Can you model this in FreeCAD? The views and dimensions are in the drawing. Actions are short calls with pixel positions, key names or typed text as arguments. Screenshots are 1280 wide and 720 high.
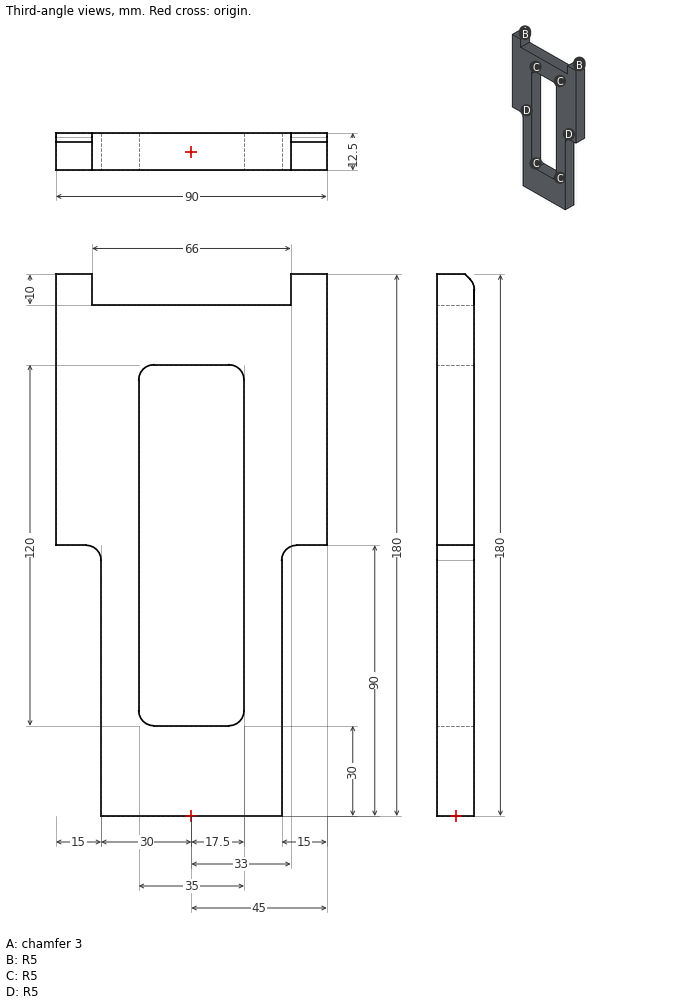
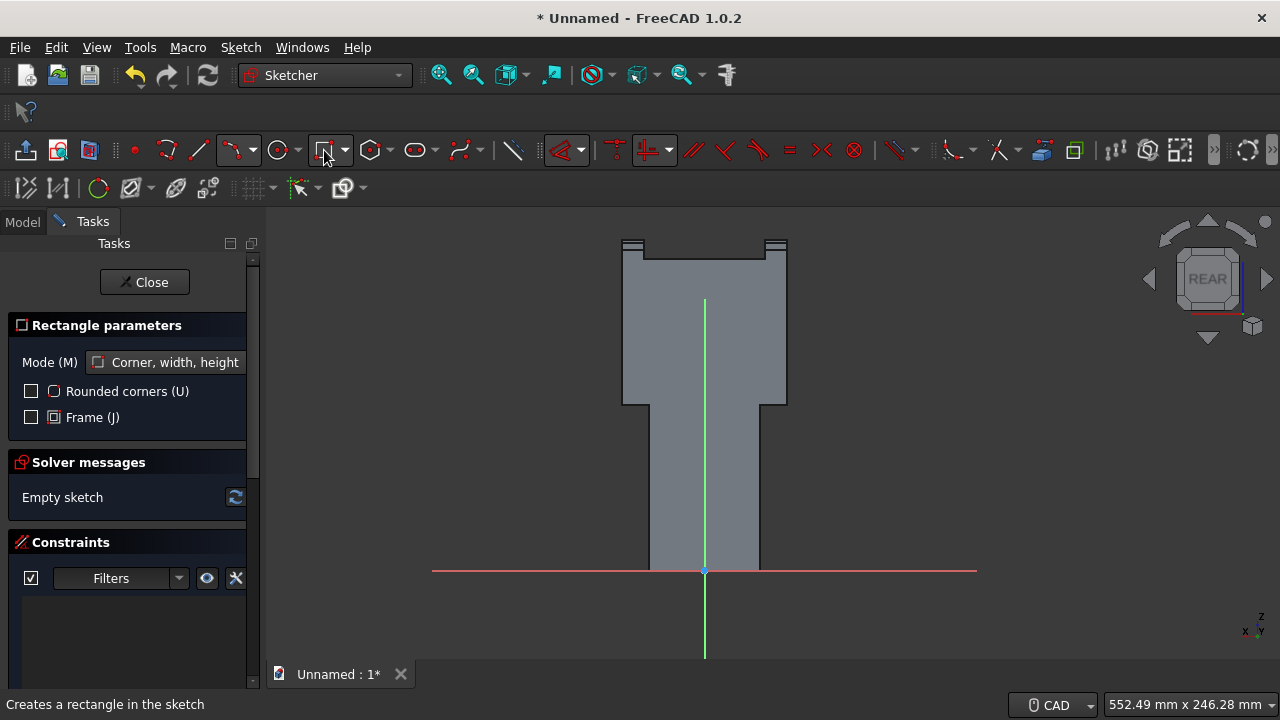
click(672, 295)
move(737, 516)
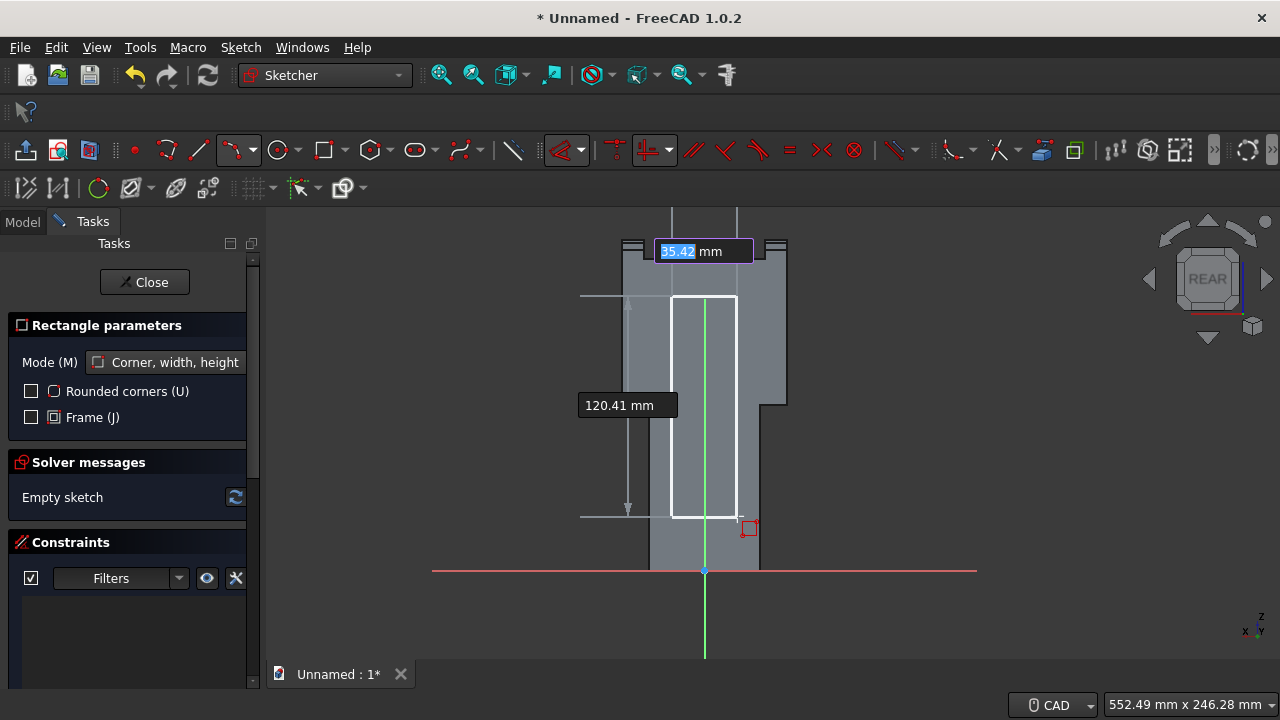
text(35)
key(Tab)
text(120)
key(Return)
key(Escape)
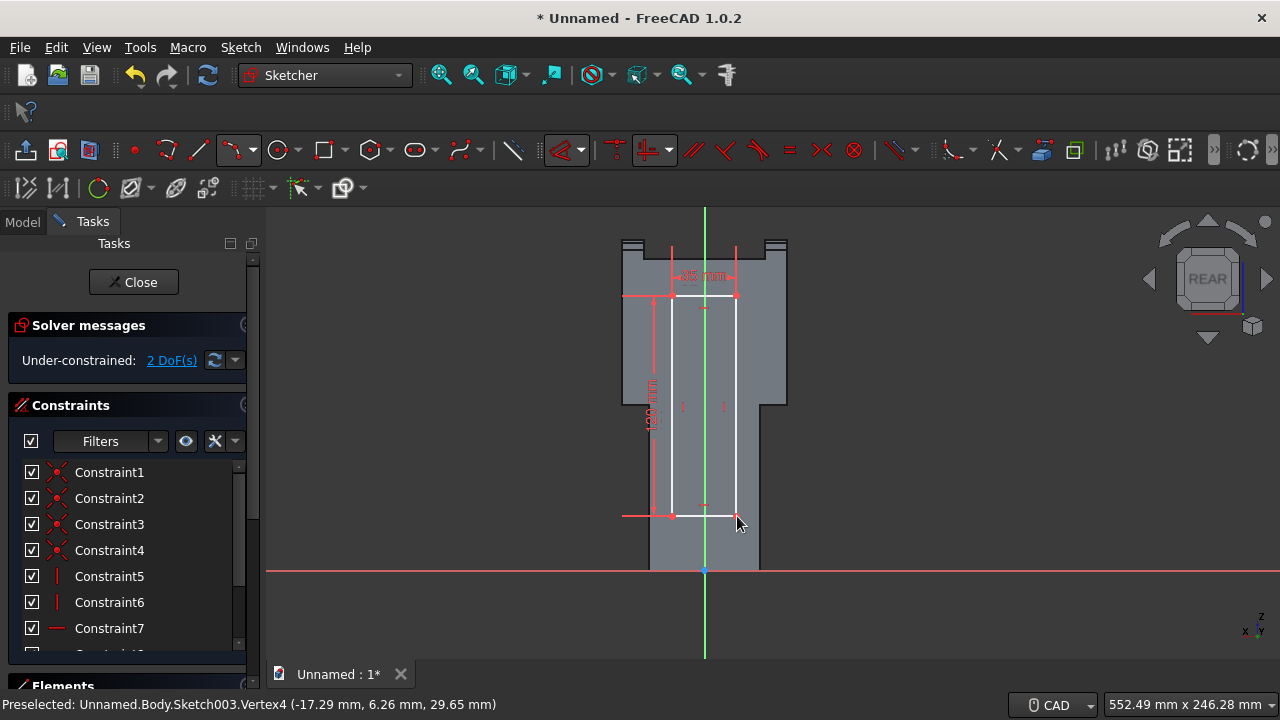
click(672, 516)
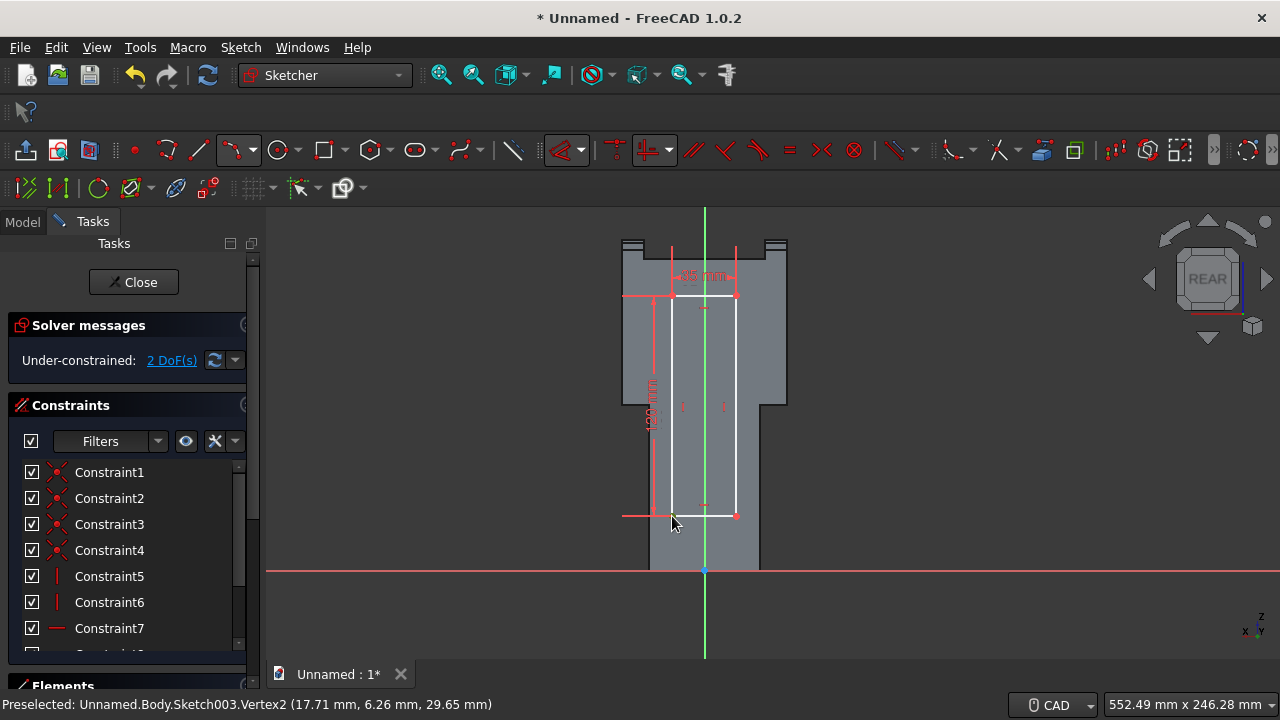
click(584, 150)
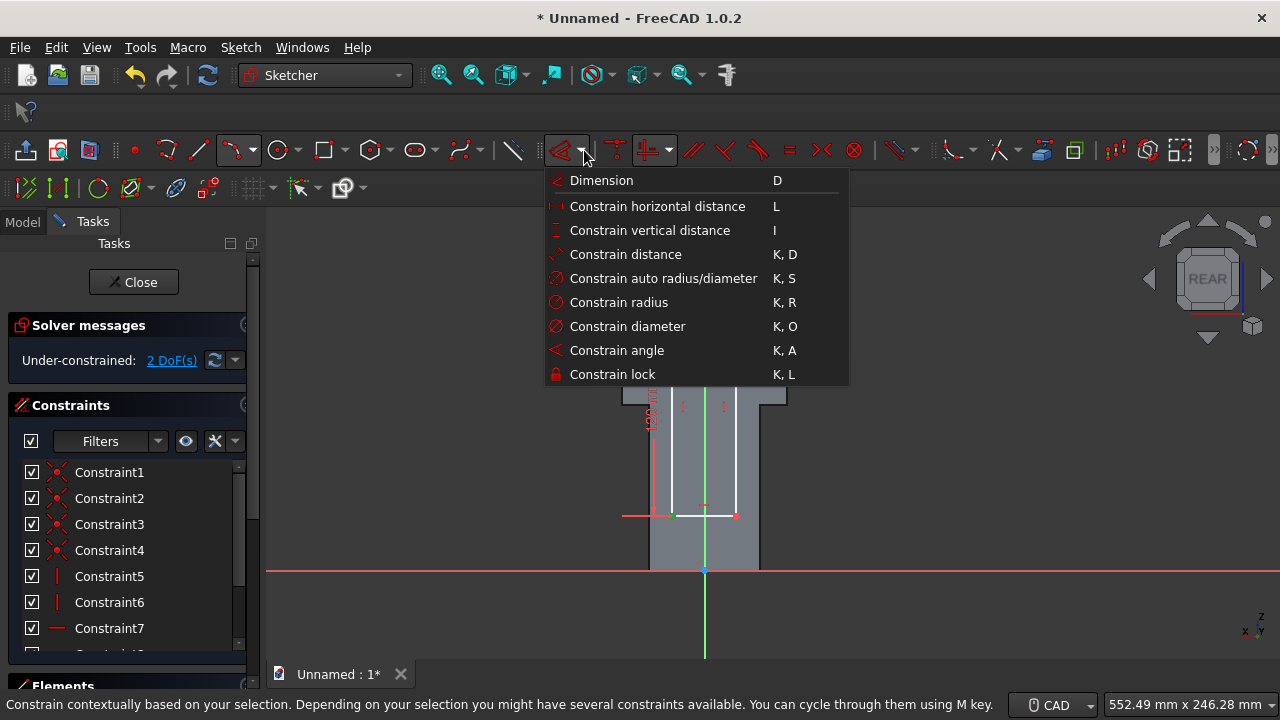
click(697, 230)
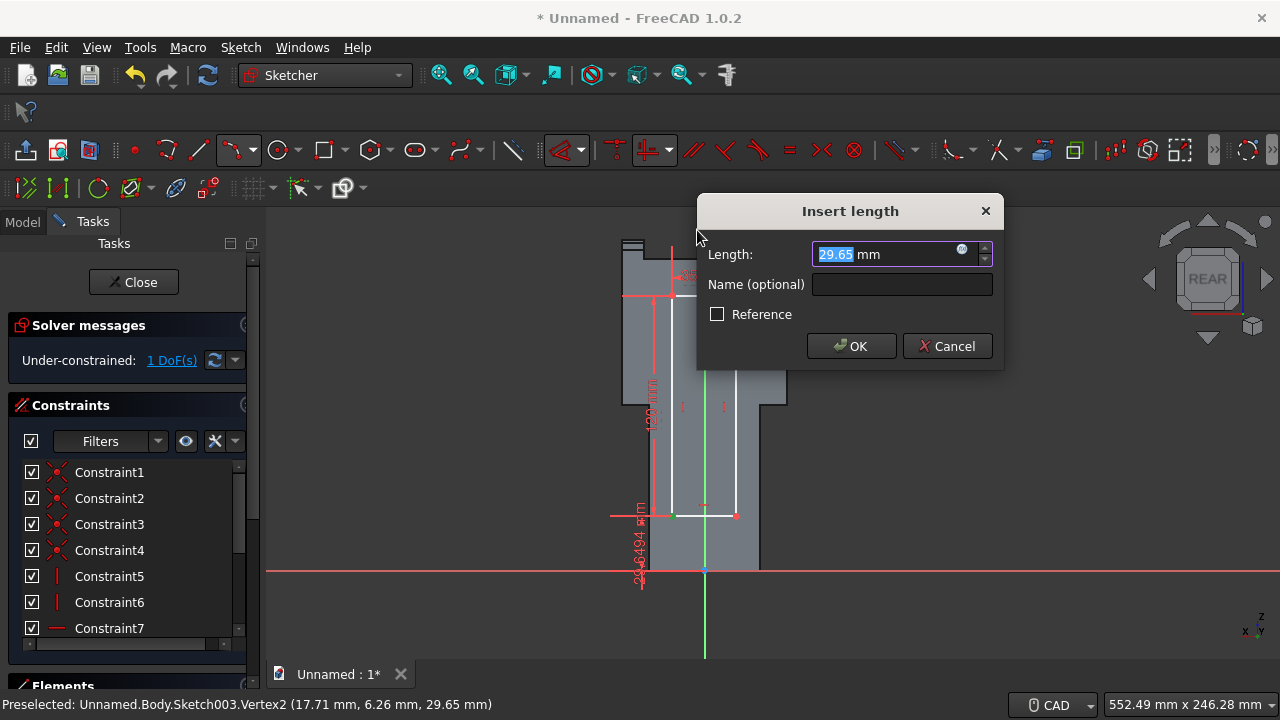
text(30)
key(Return)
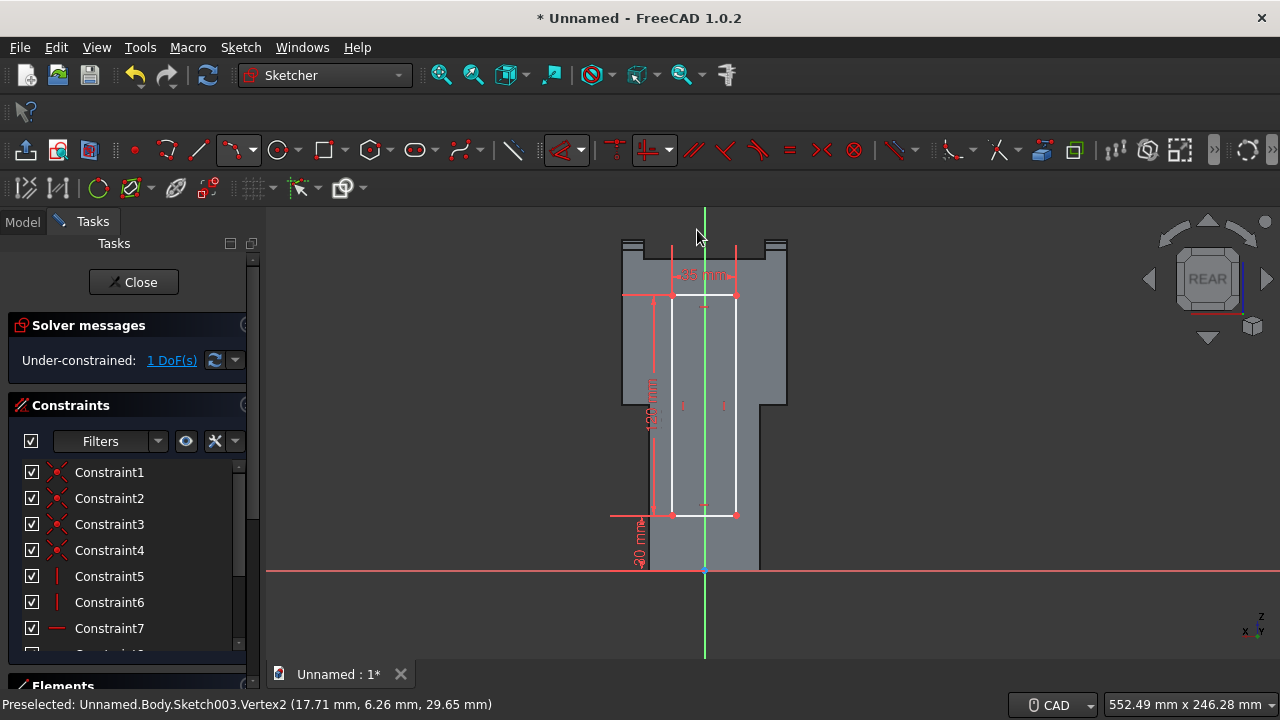
scroll(672, 295, up, 2)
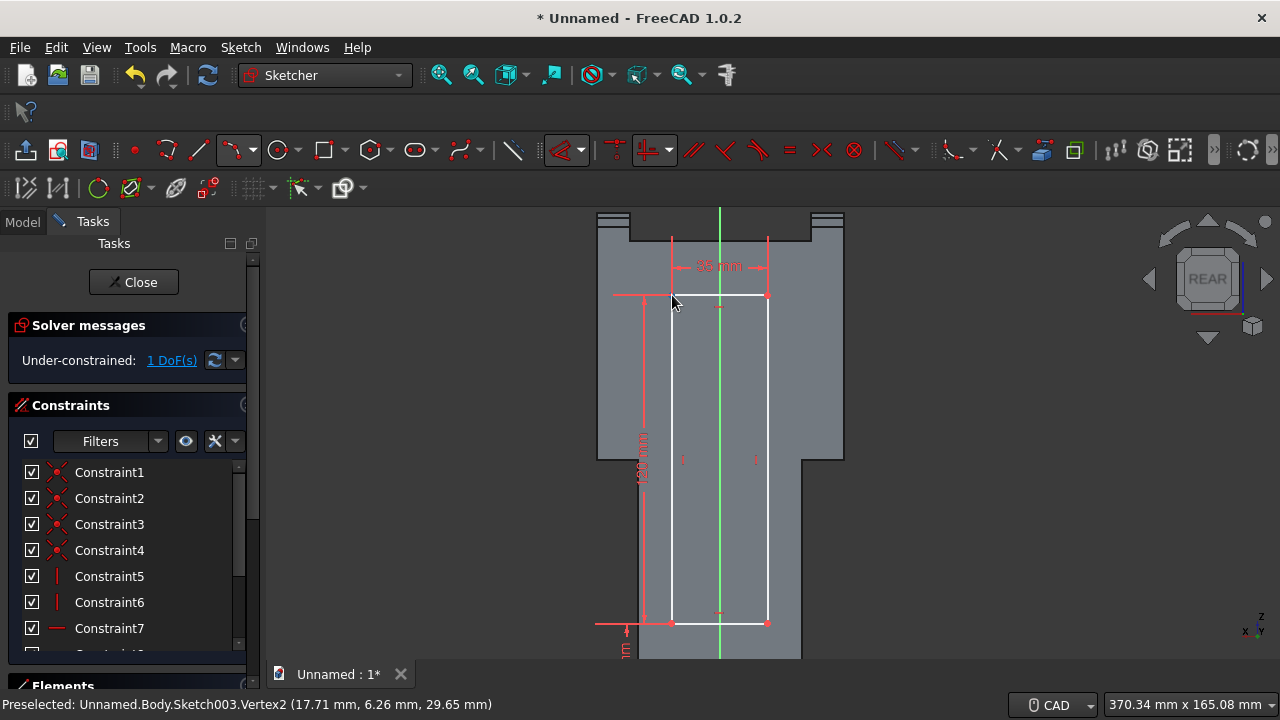
click(672, 295)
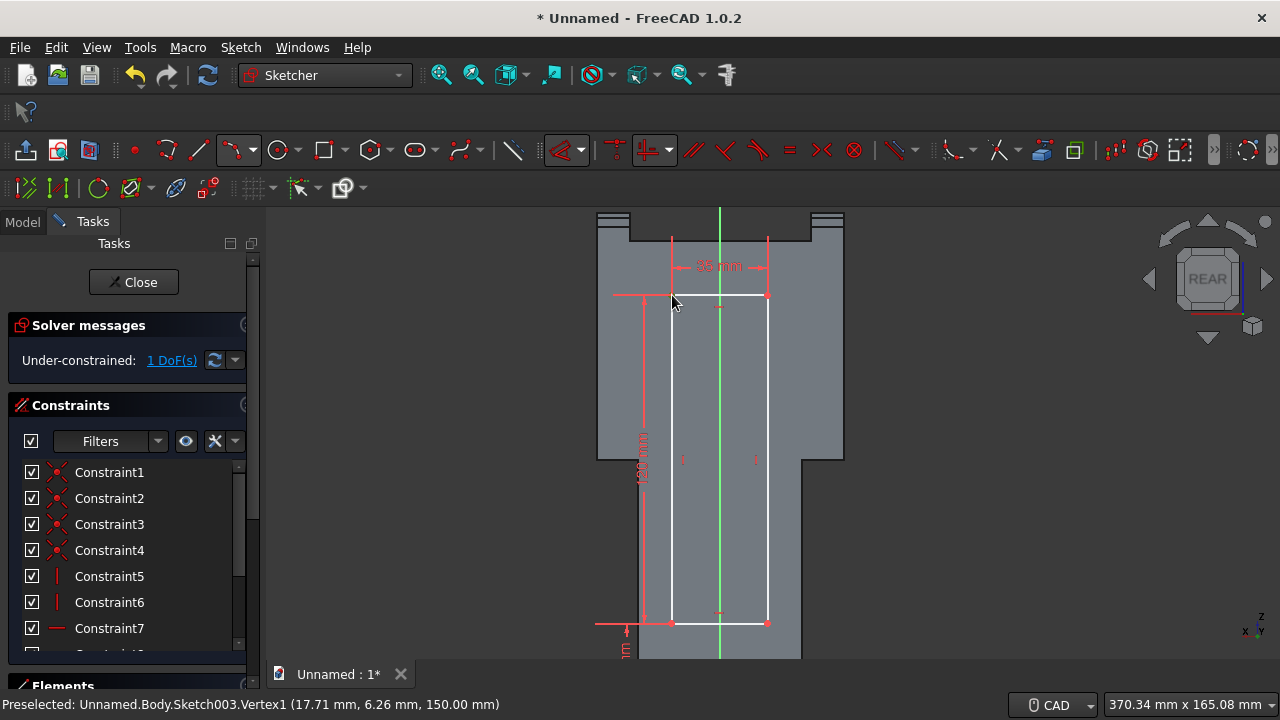
click(584, 150)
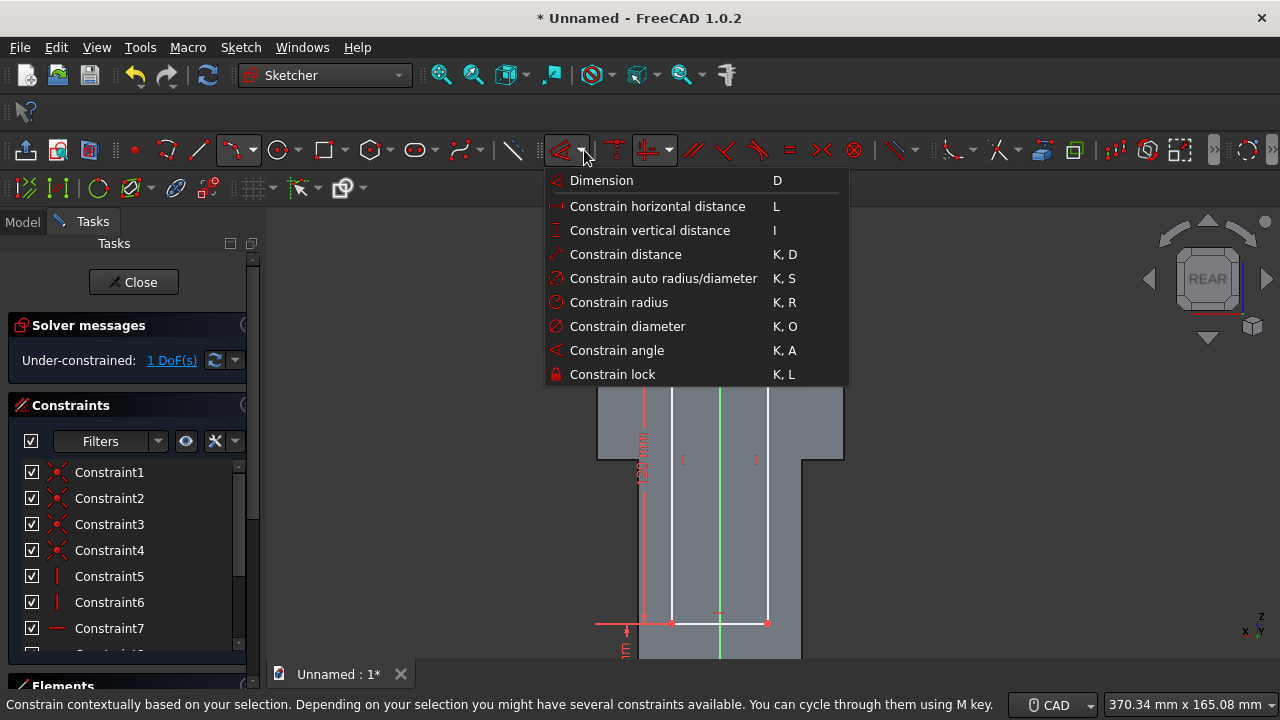
click(697, 206)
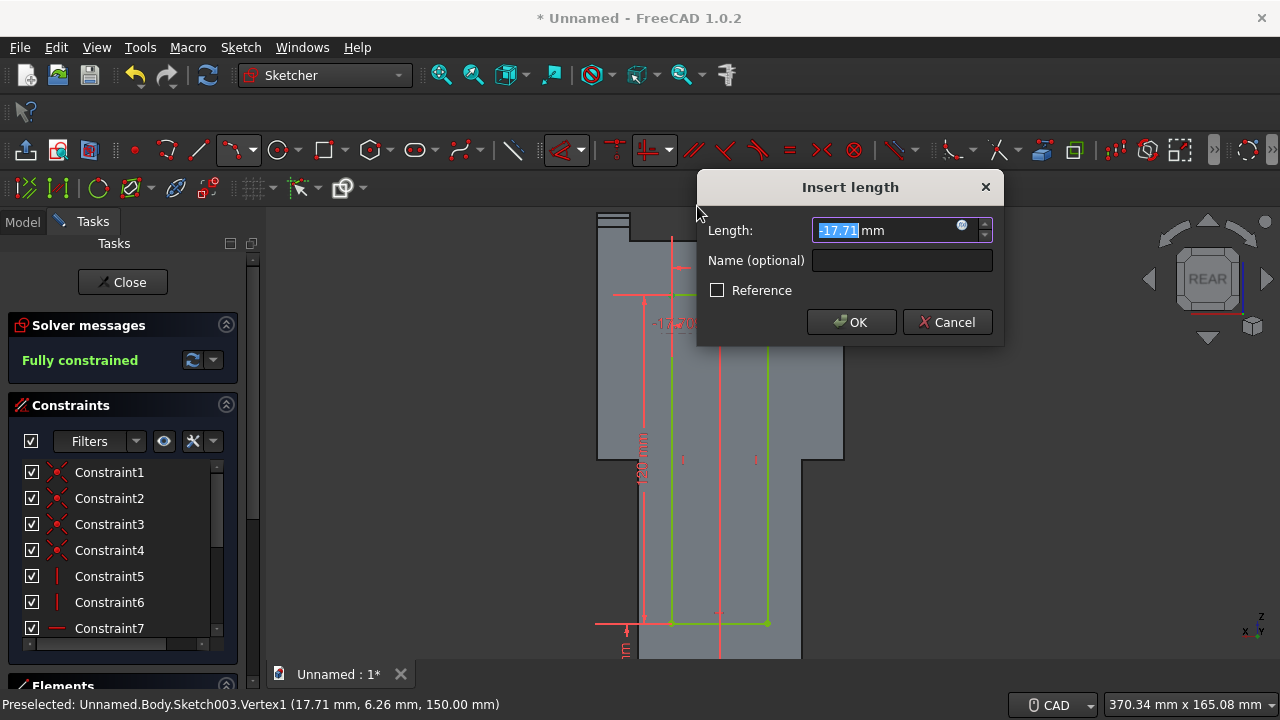
text(-17.5)
key(Return)